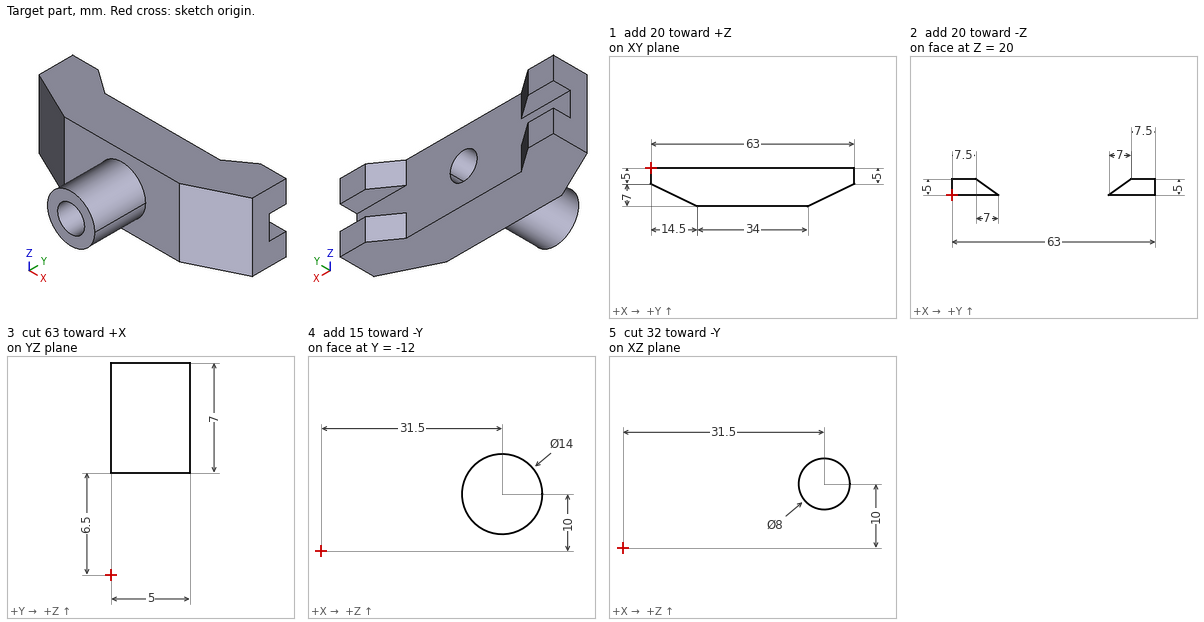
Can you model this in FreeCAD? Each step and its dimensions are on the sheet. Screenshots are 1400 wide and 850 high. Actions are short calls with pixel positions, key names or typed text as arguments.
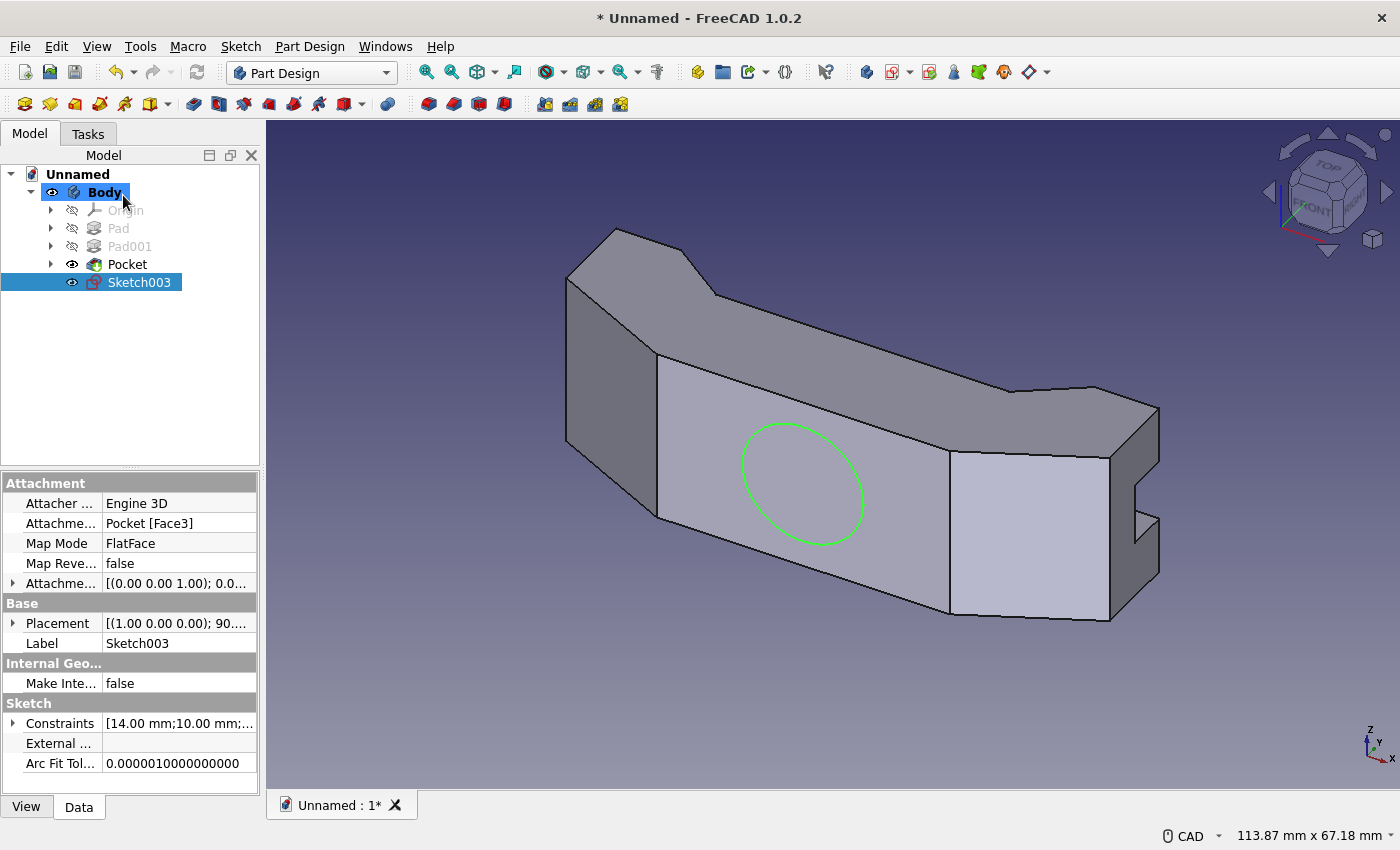
click(25, 104)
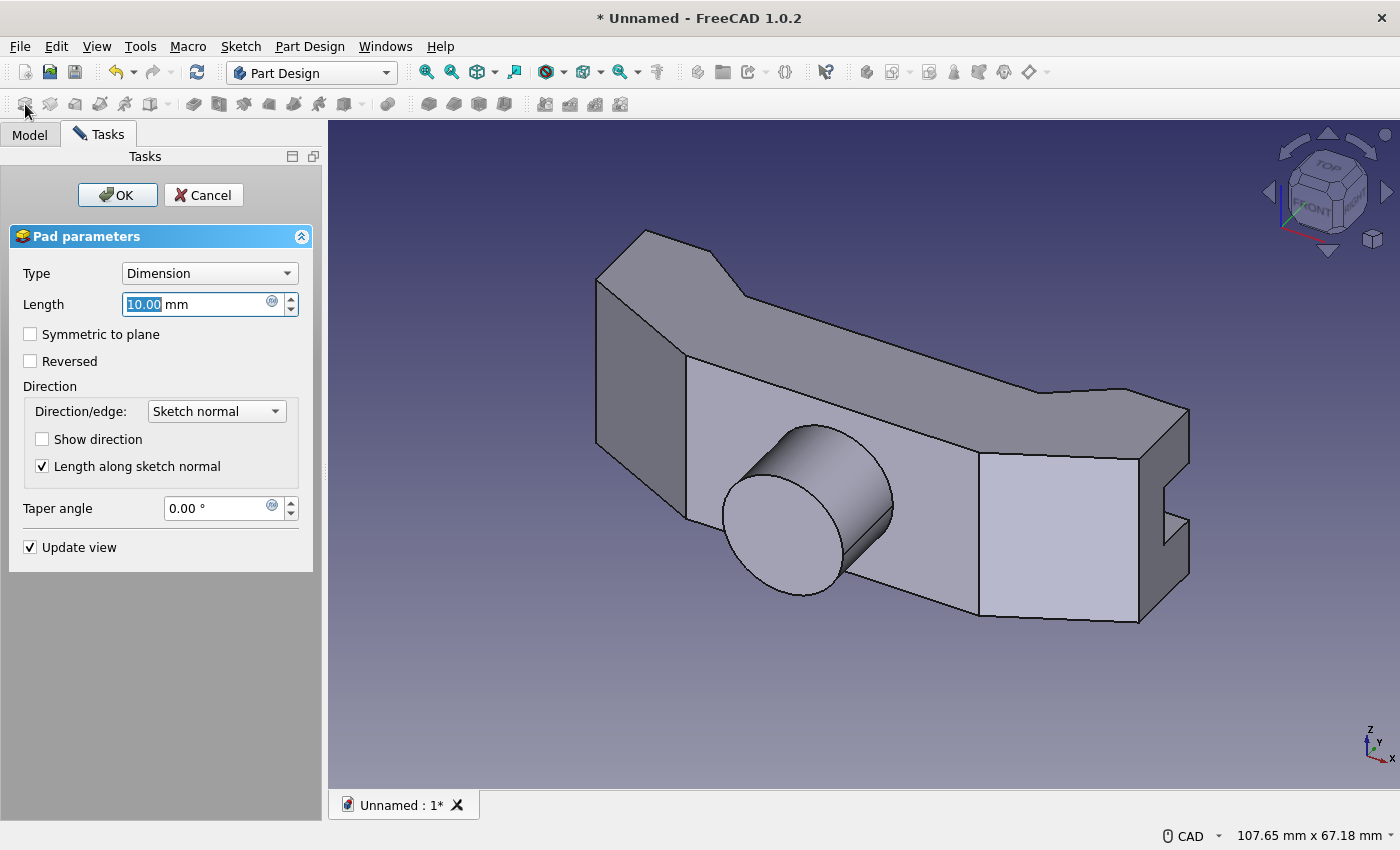
text(15)
key(Tab)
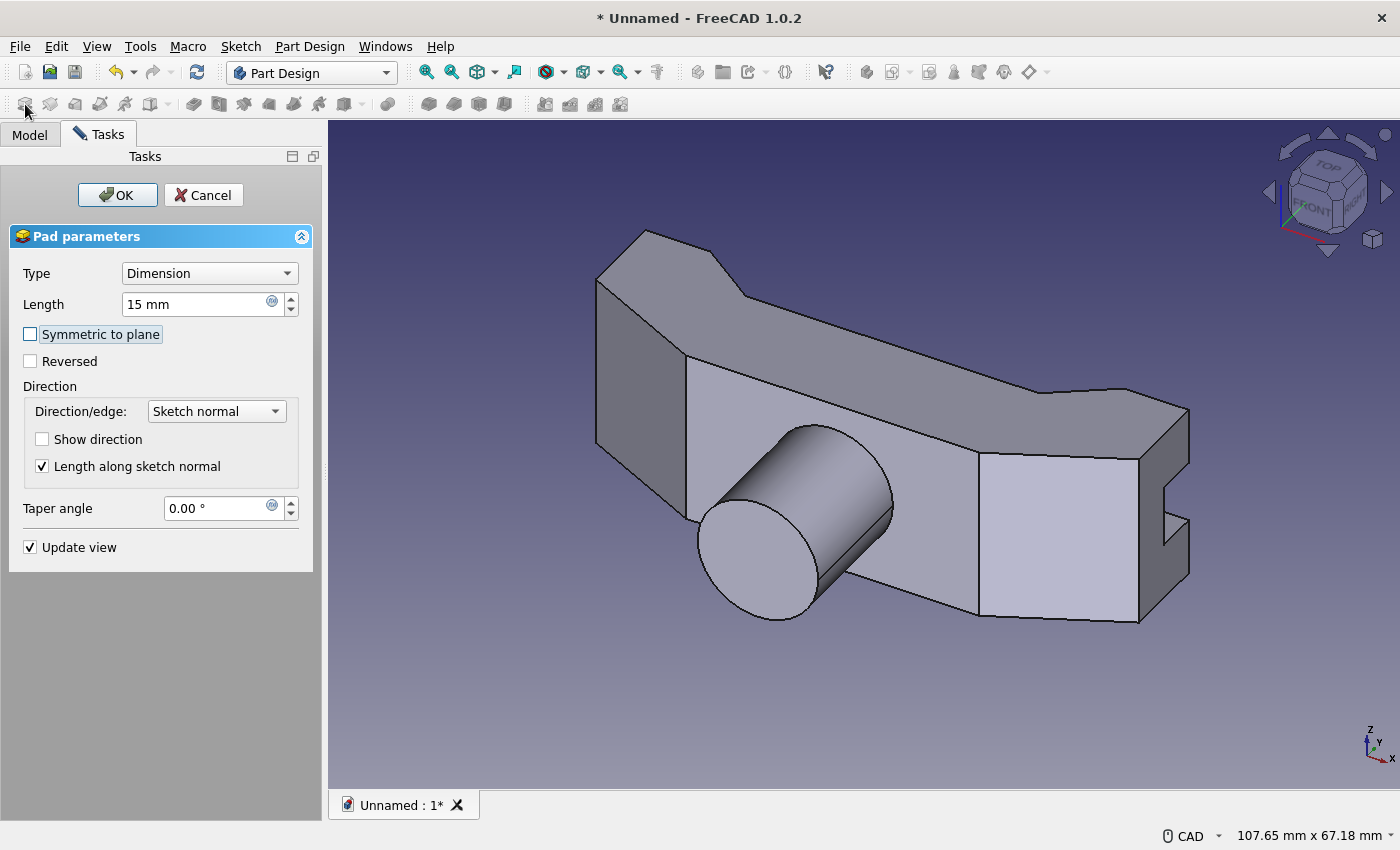
click(118, 195)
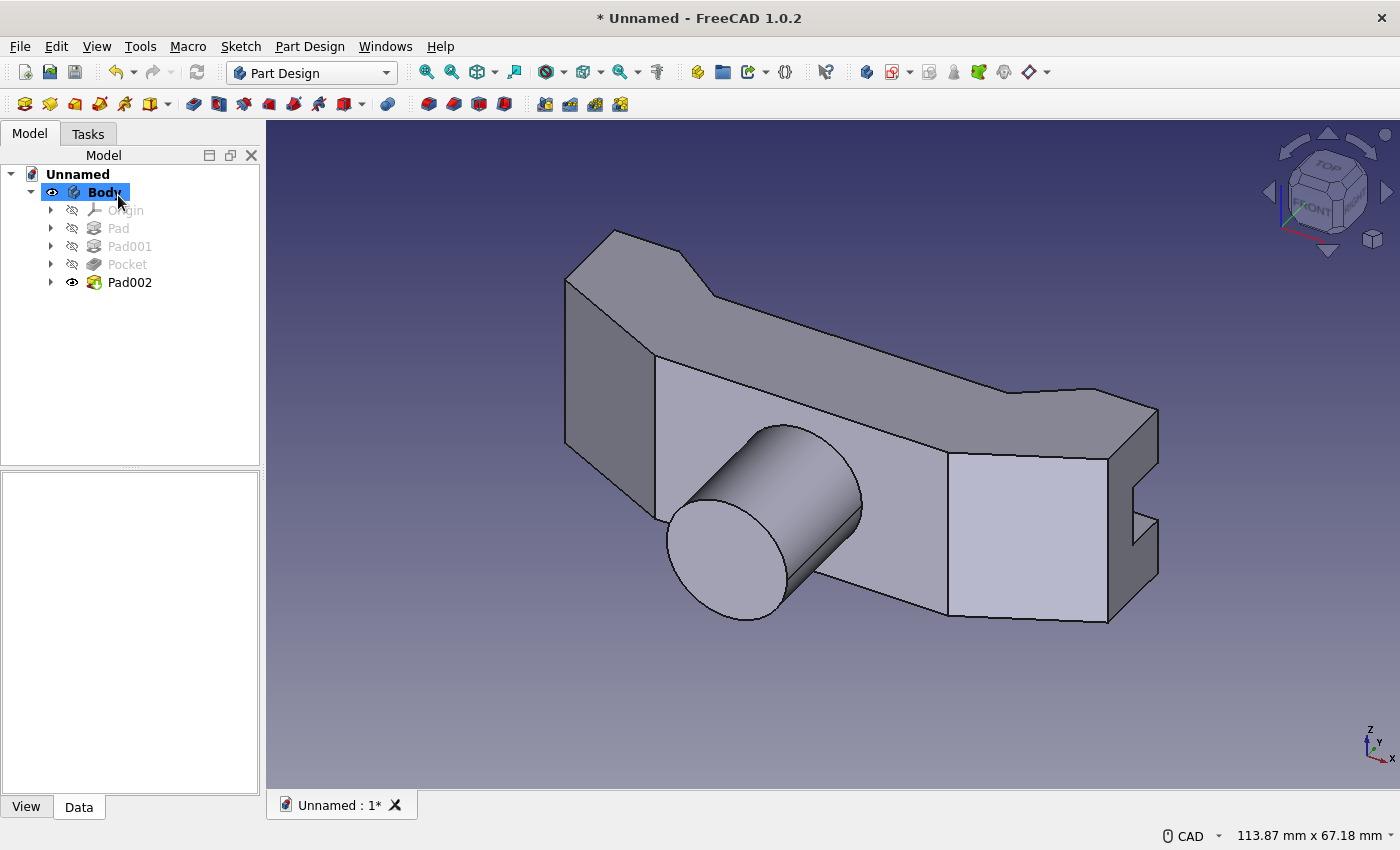
click(892, 72)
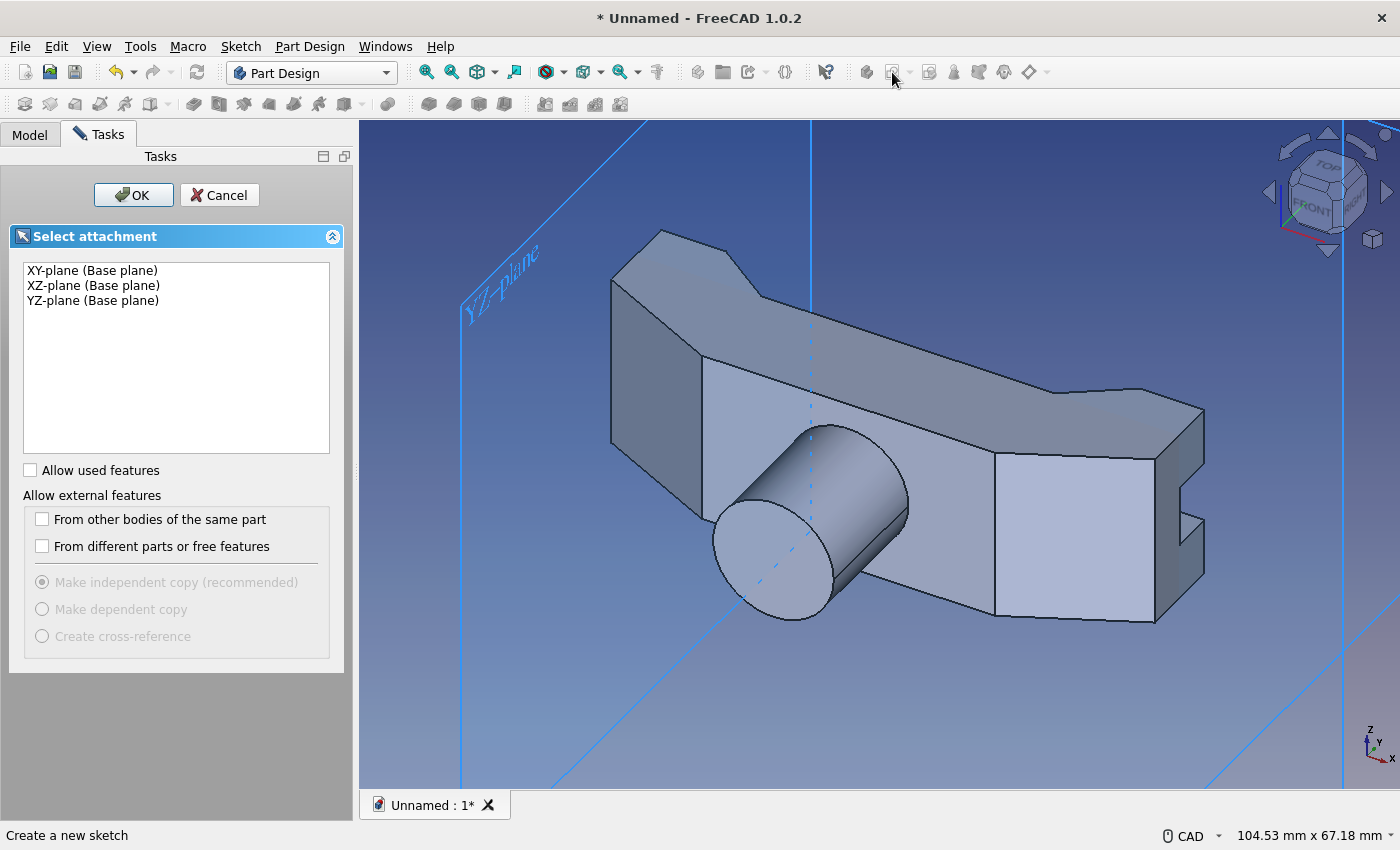
click(84, 286)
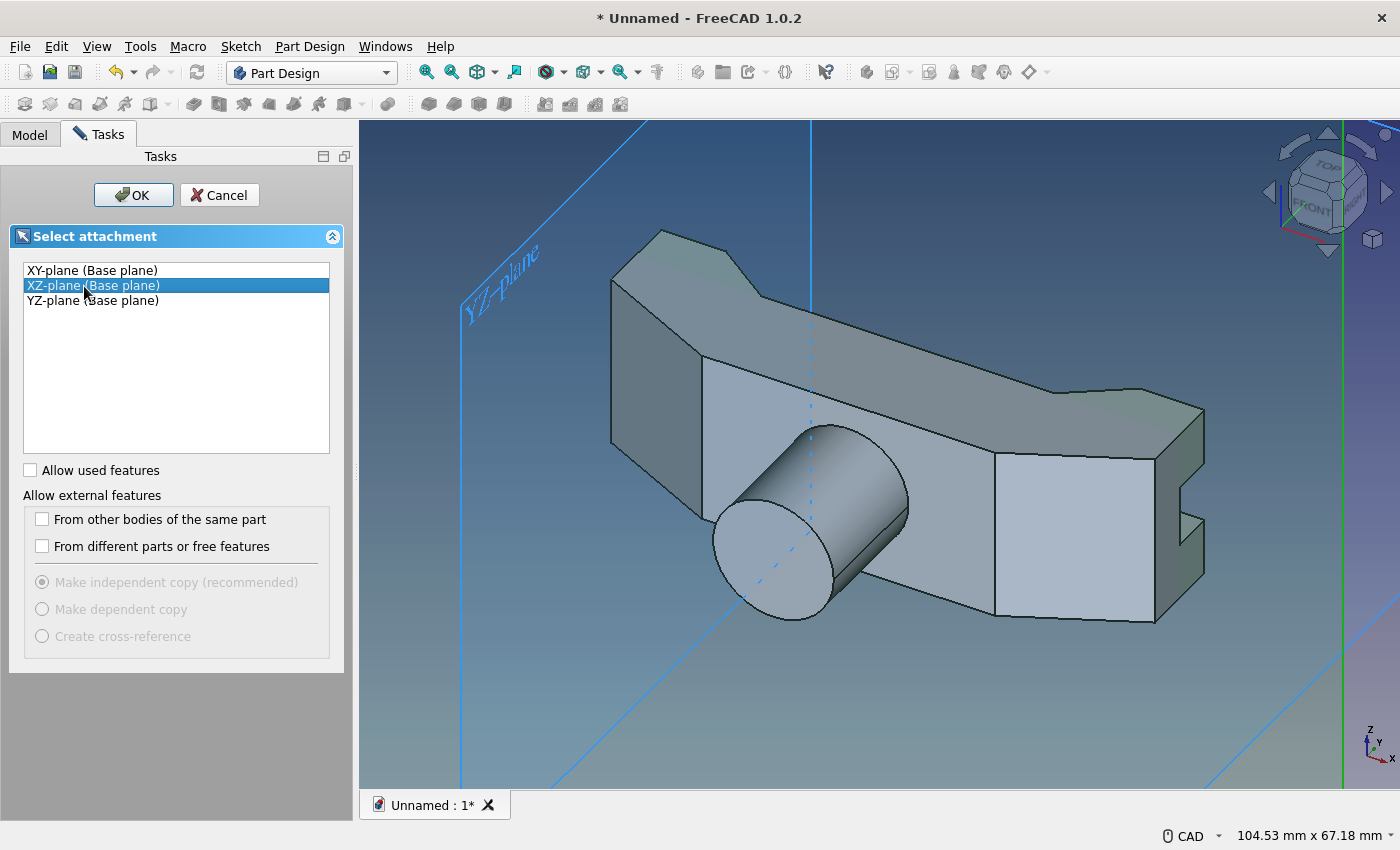
click(134, 195)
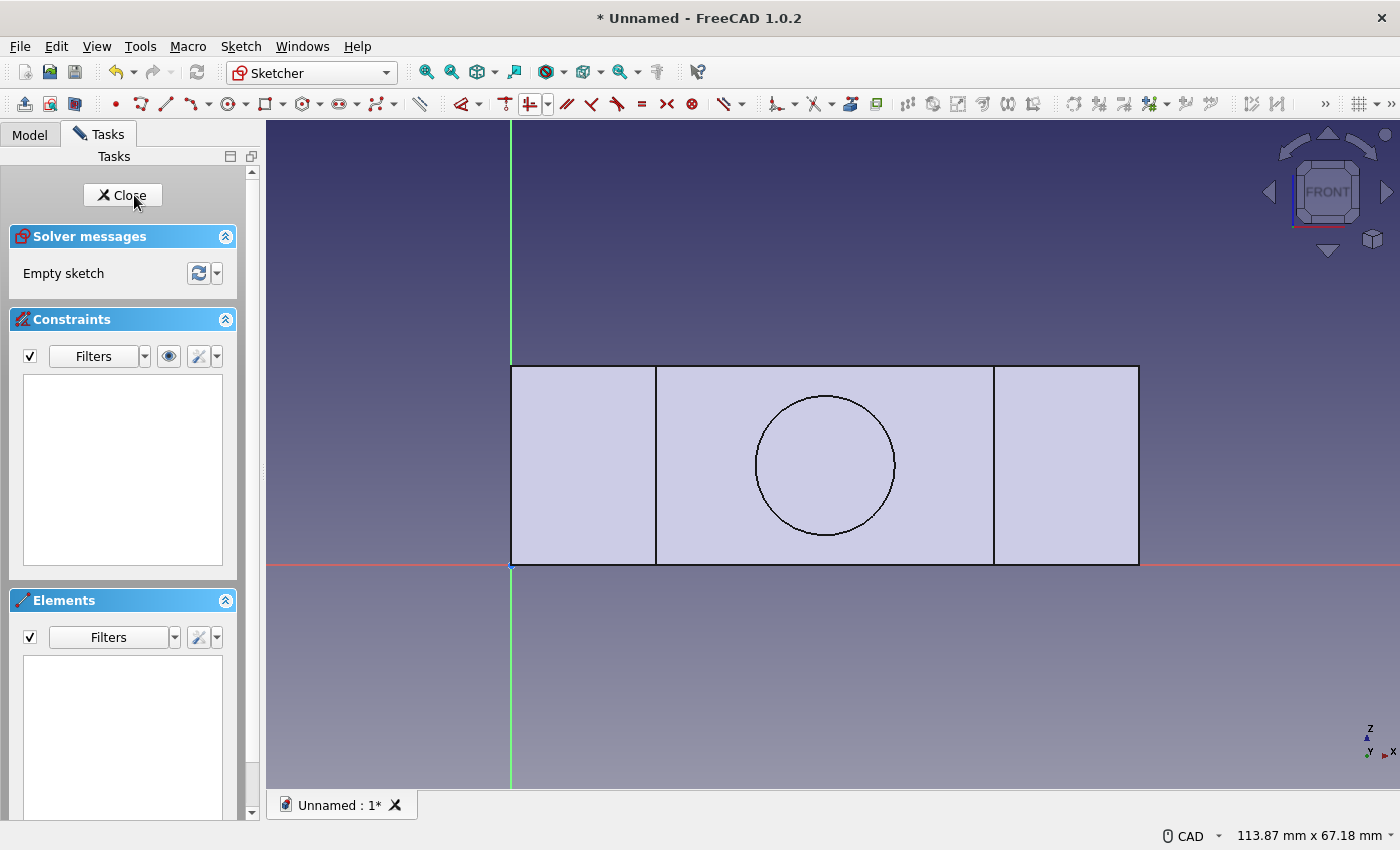
click(75, 104)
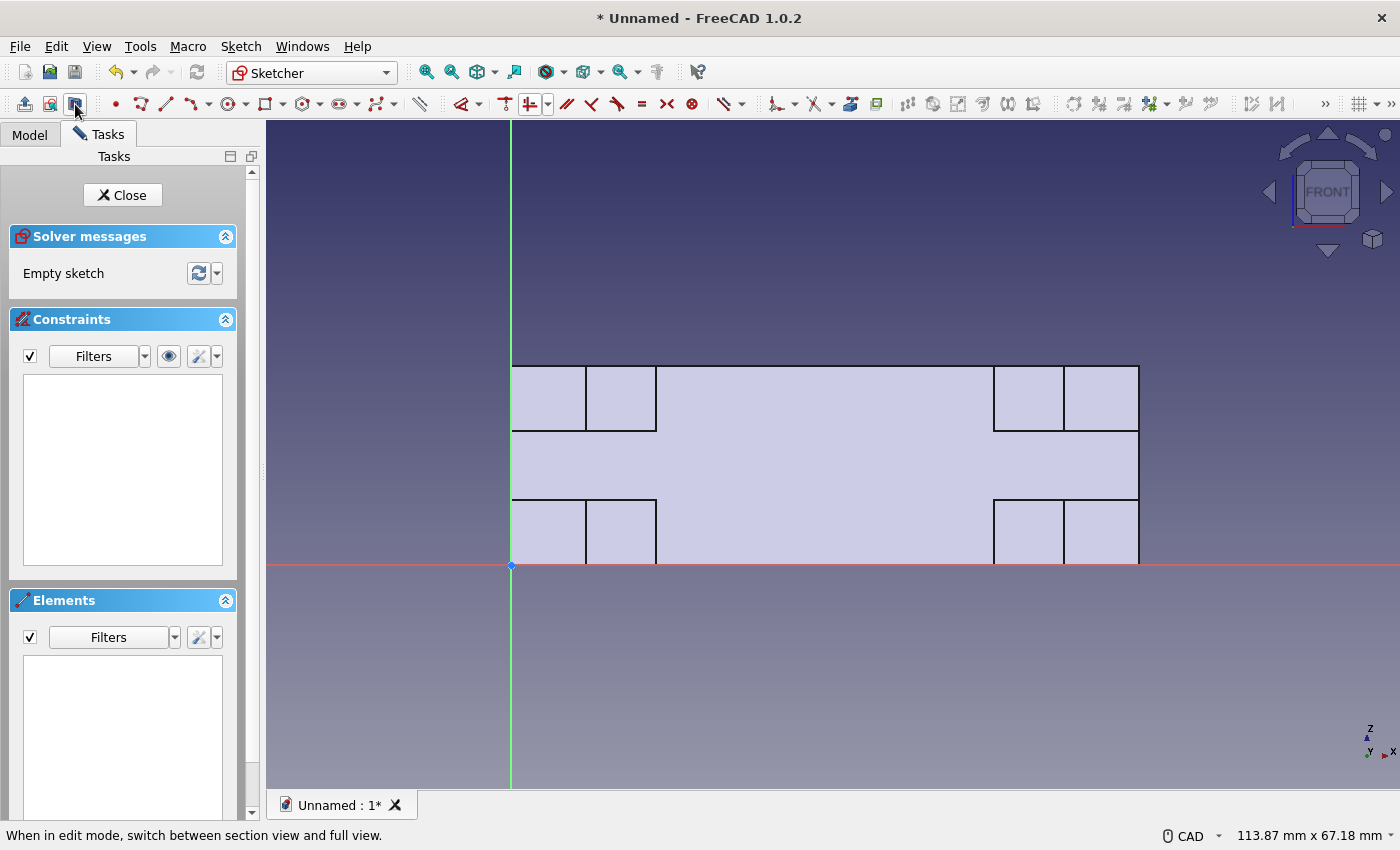
scroll(840, 468, up, 8)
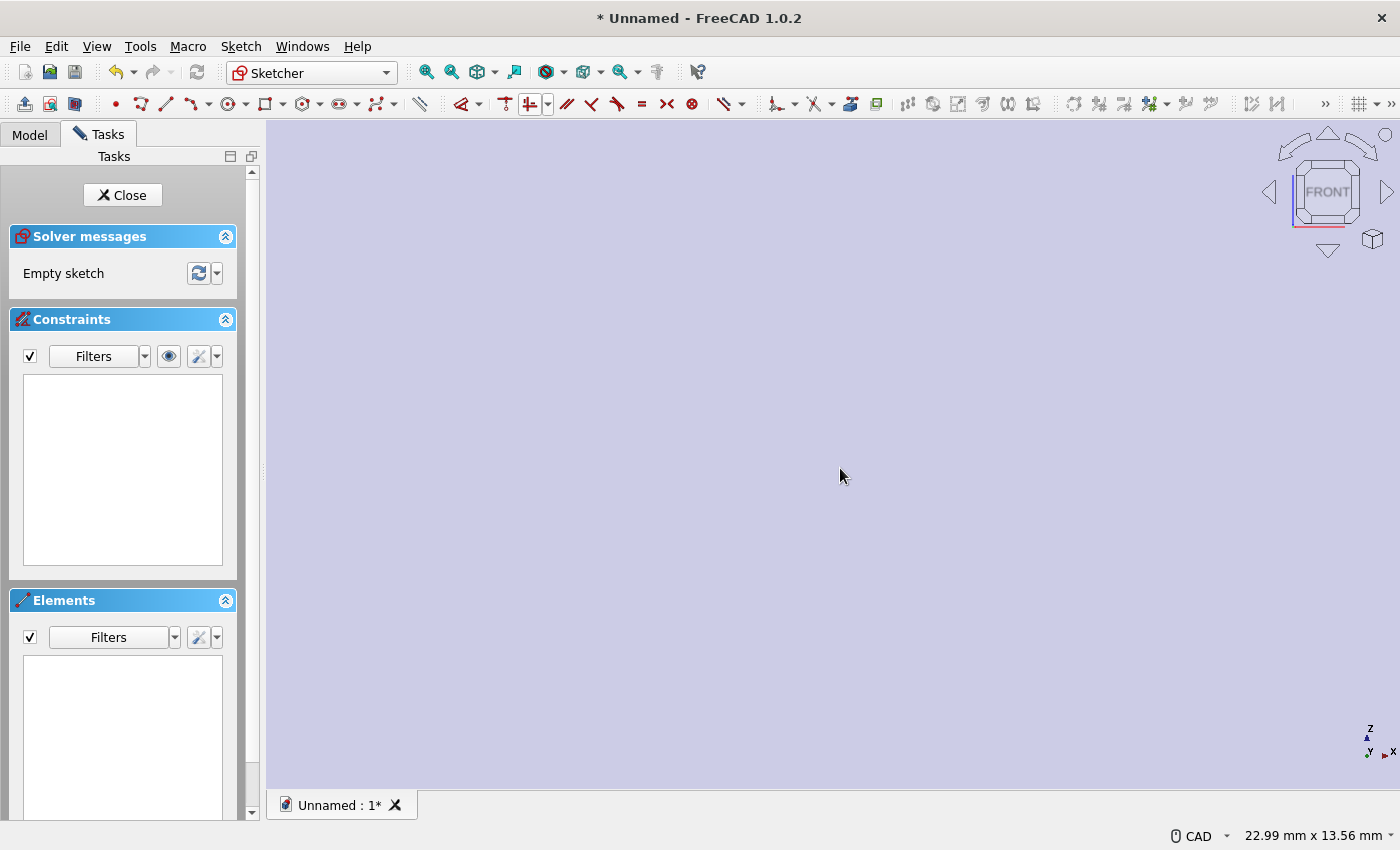
click(228, 104)